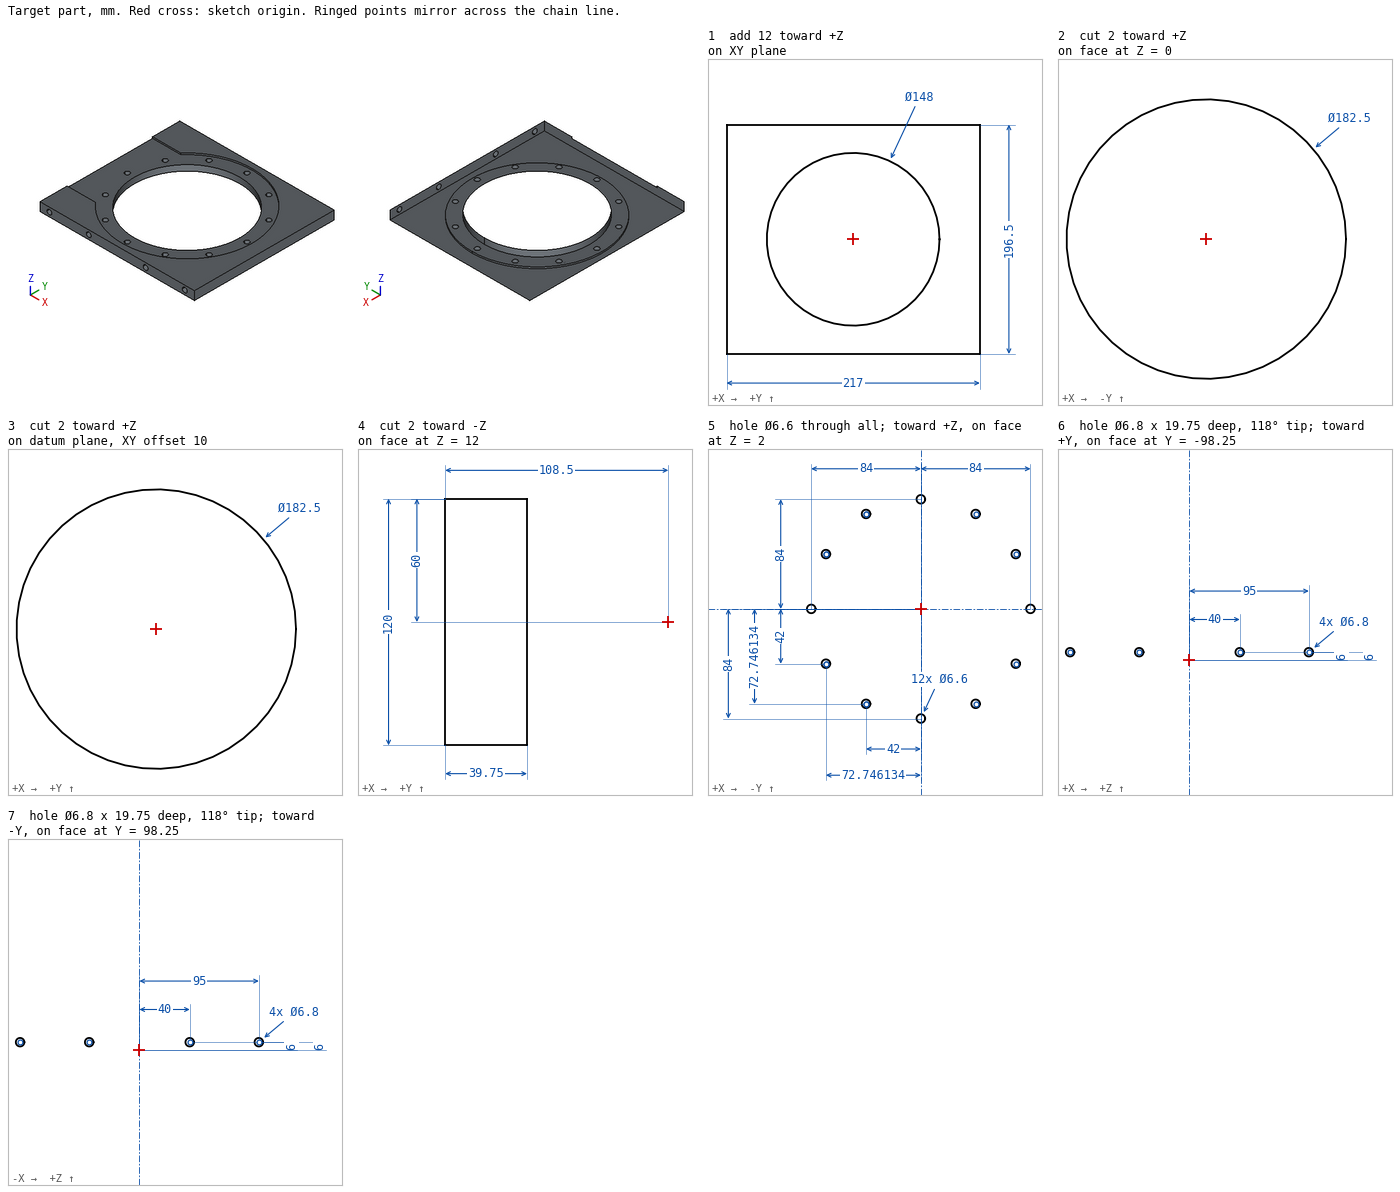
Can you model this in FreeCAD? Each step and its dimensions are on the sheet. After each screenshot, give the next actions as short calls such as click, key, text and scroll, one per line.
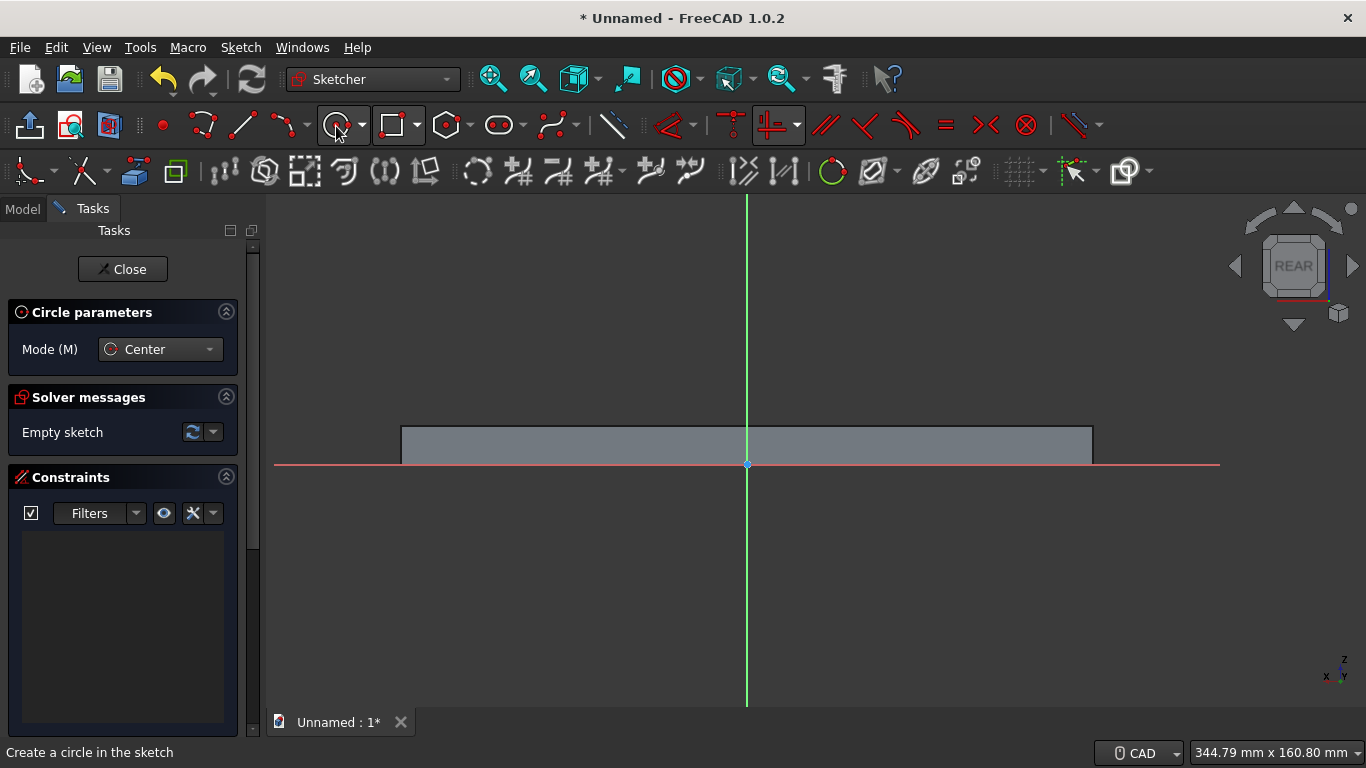
scroll(1050, 446, up, 4)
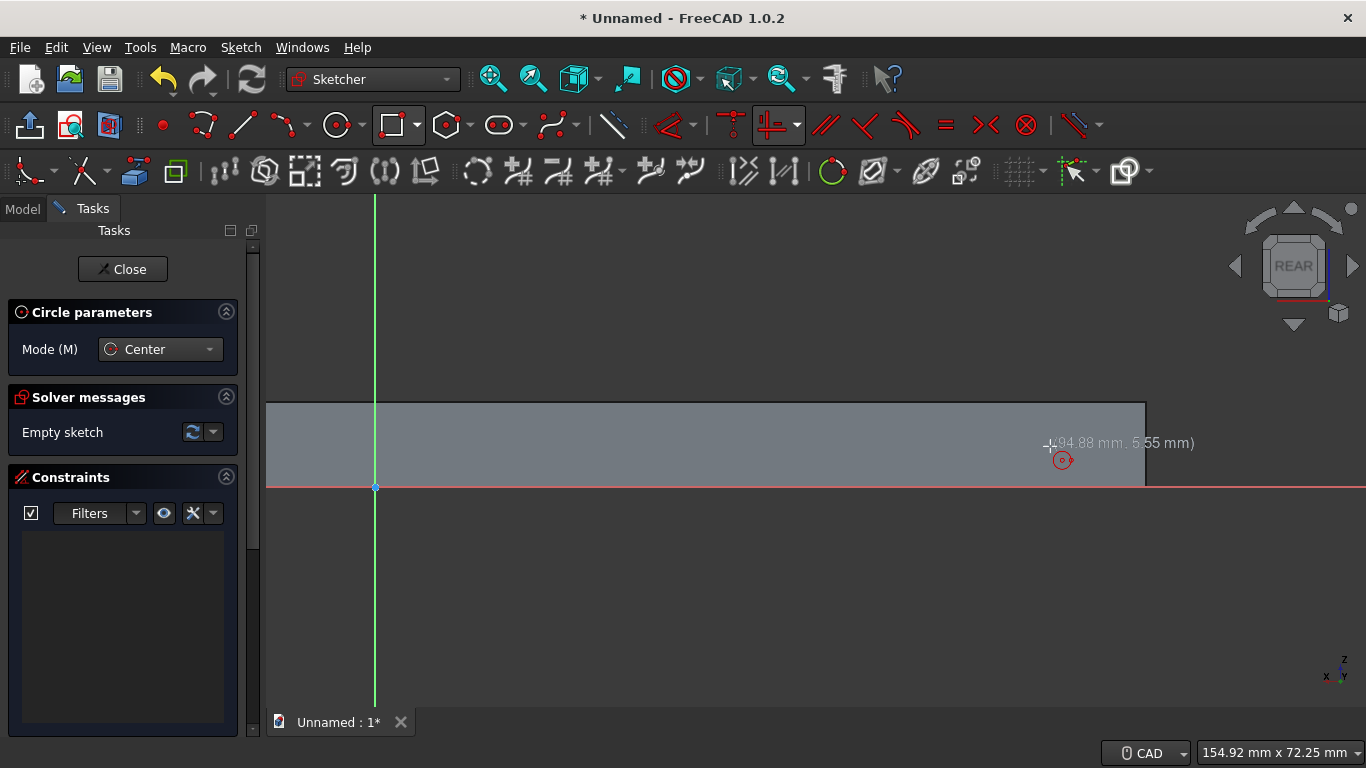
click(1050, 444)
click(1067, 427)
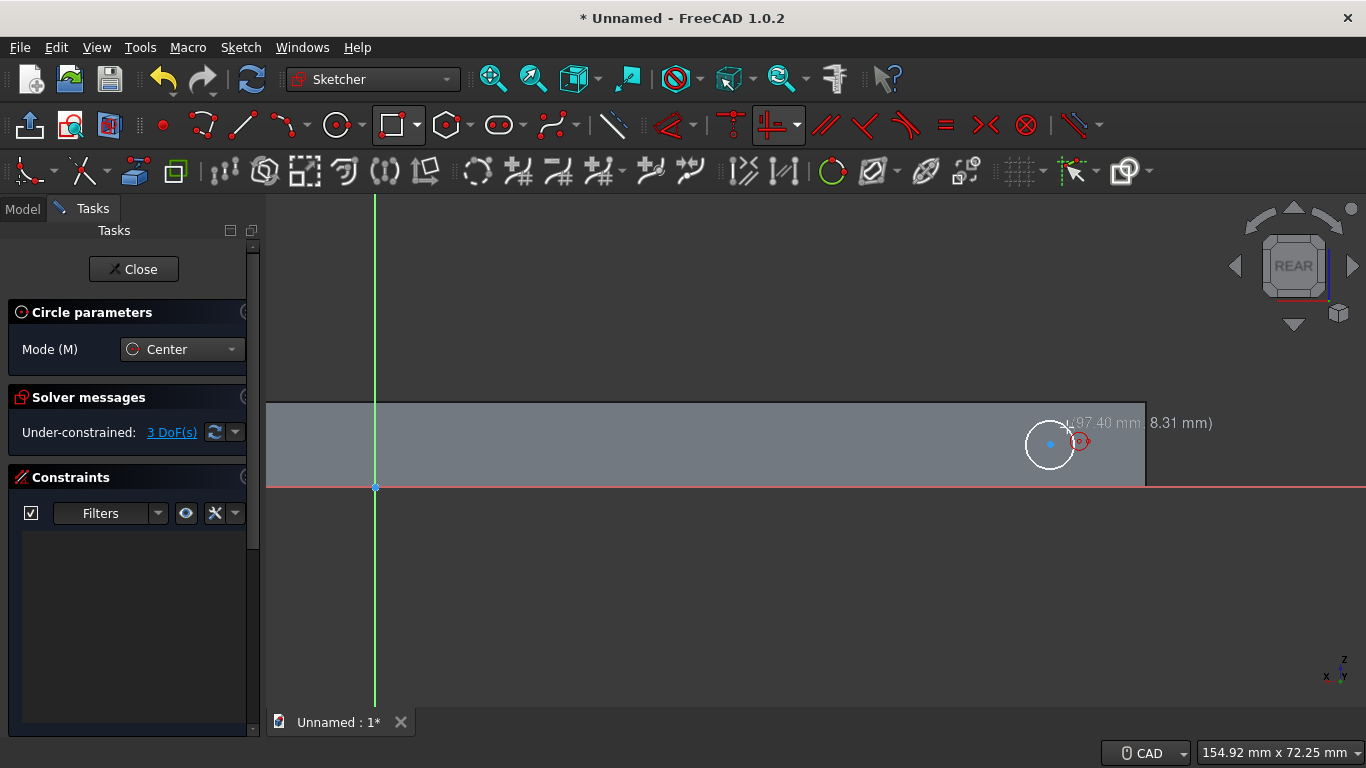
click(659, 444)
click(677, 427)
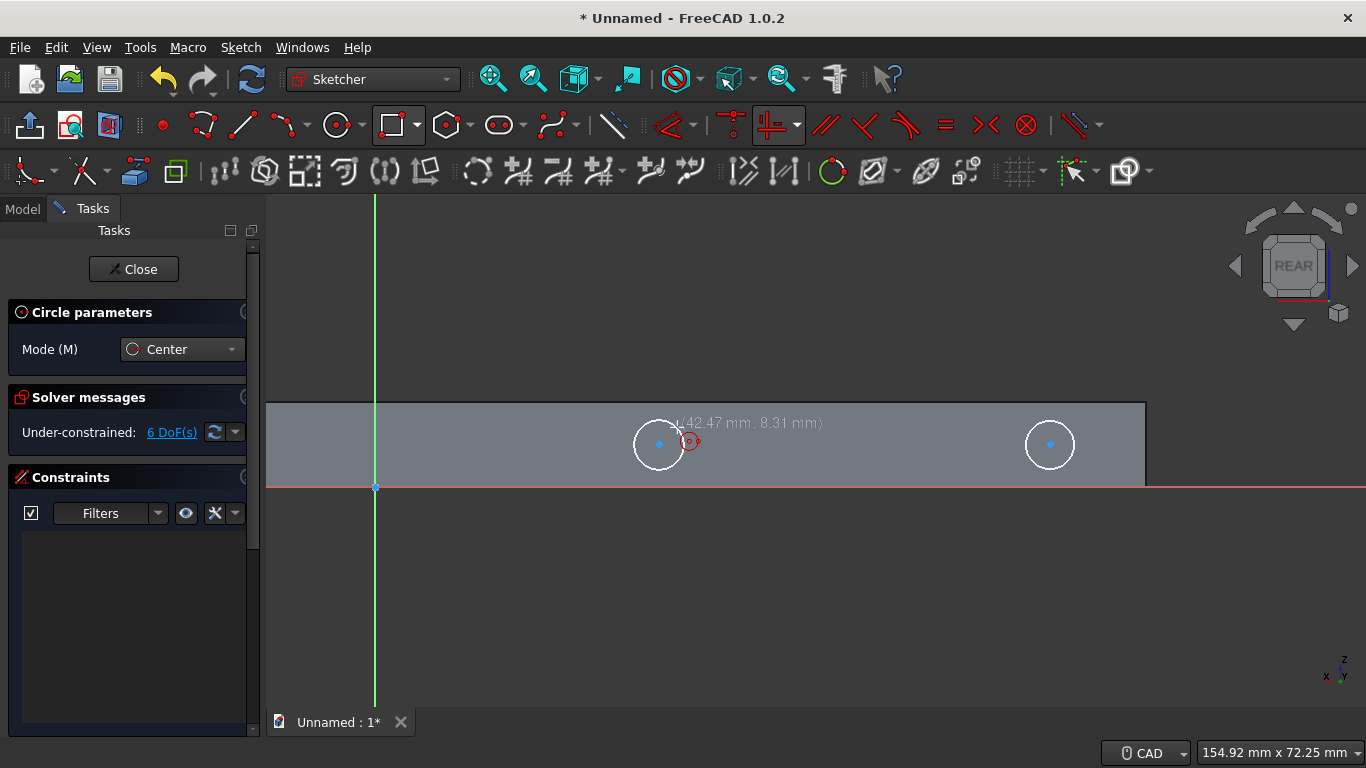
scroll(1051, 448, down, 4)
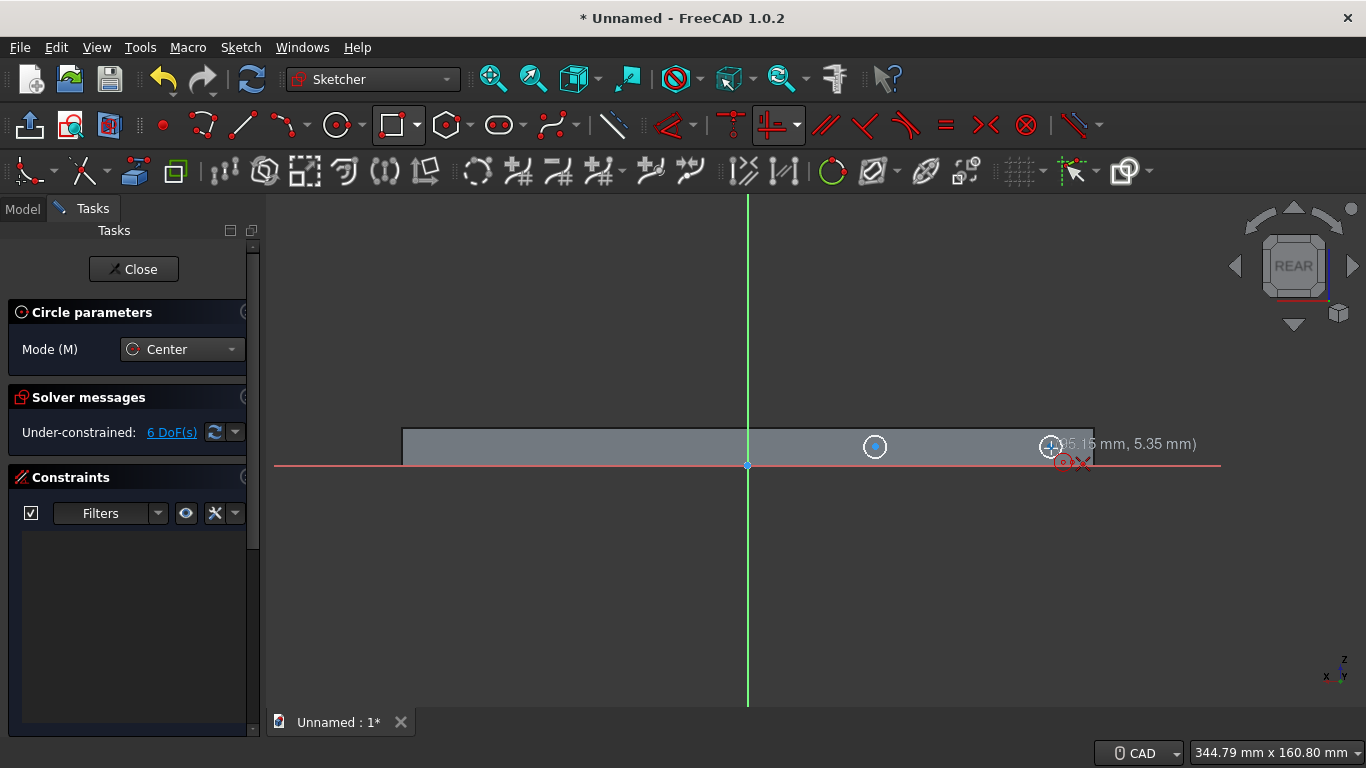
scroll(620, 447, up, 4)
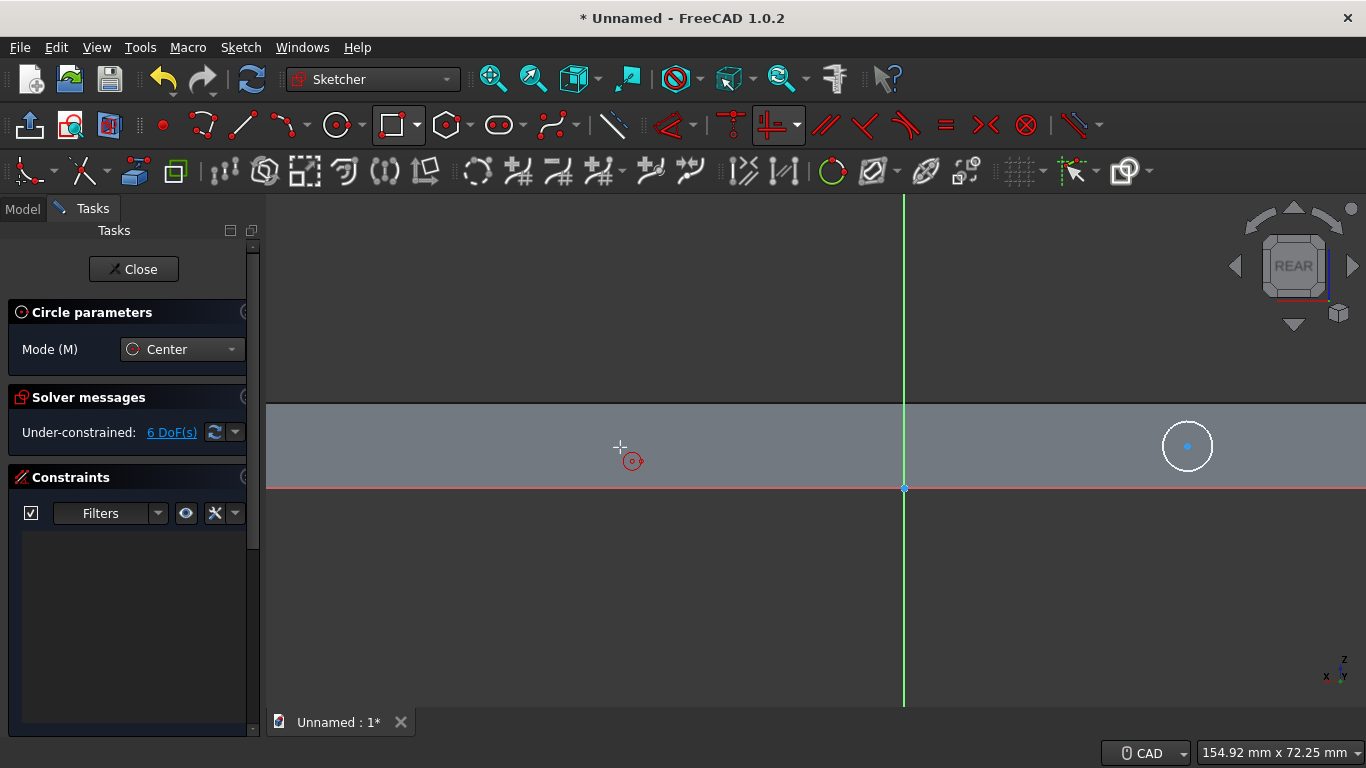
click(620, 446)
click(637, 429)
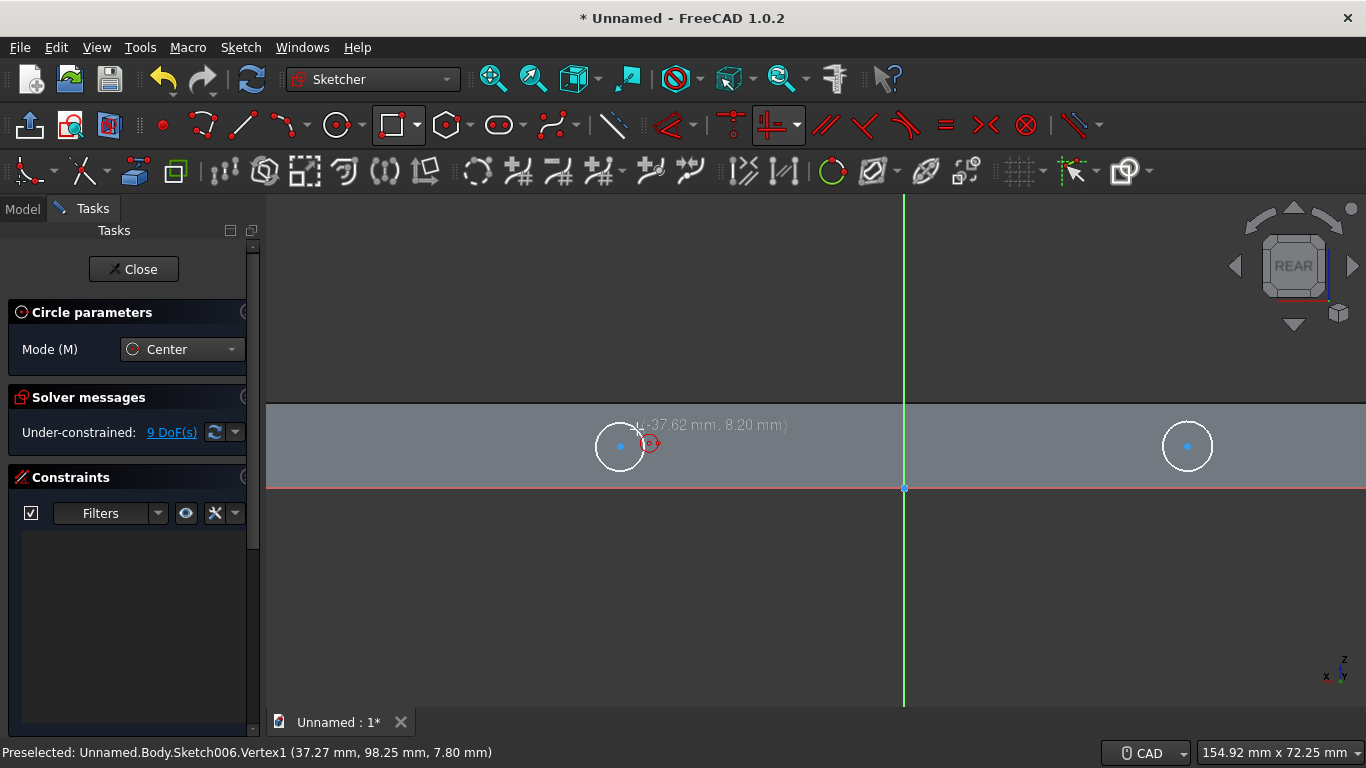
scroll(620, 447, down, 4)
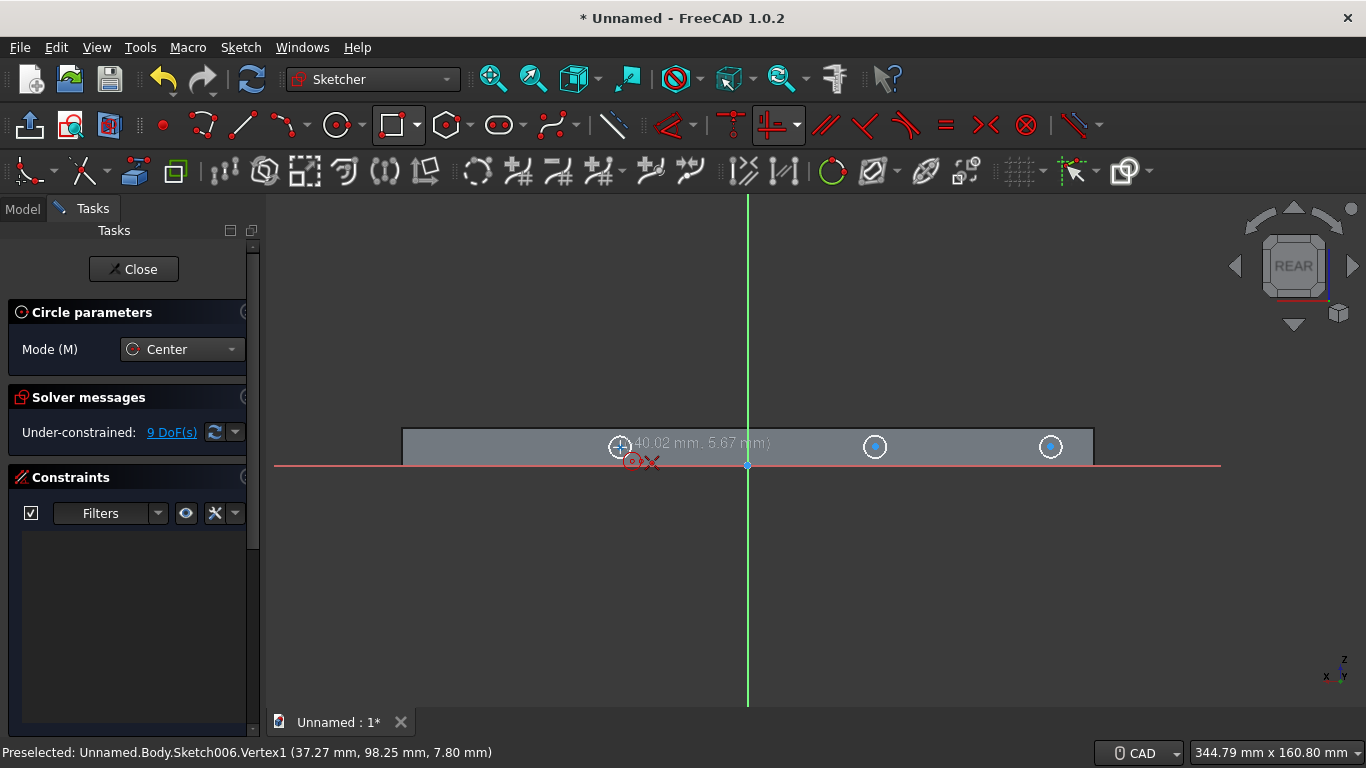
scroll(445, 447, up, 4)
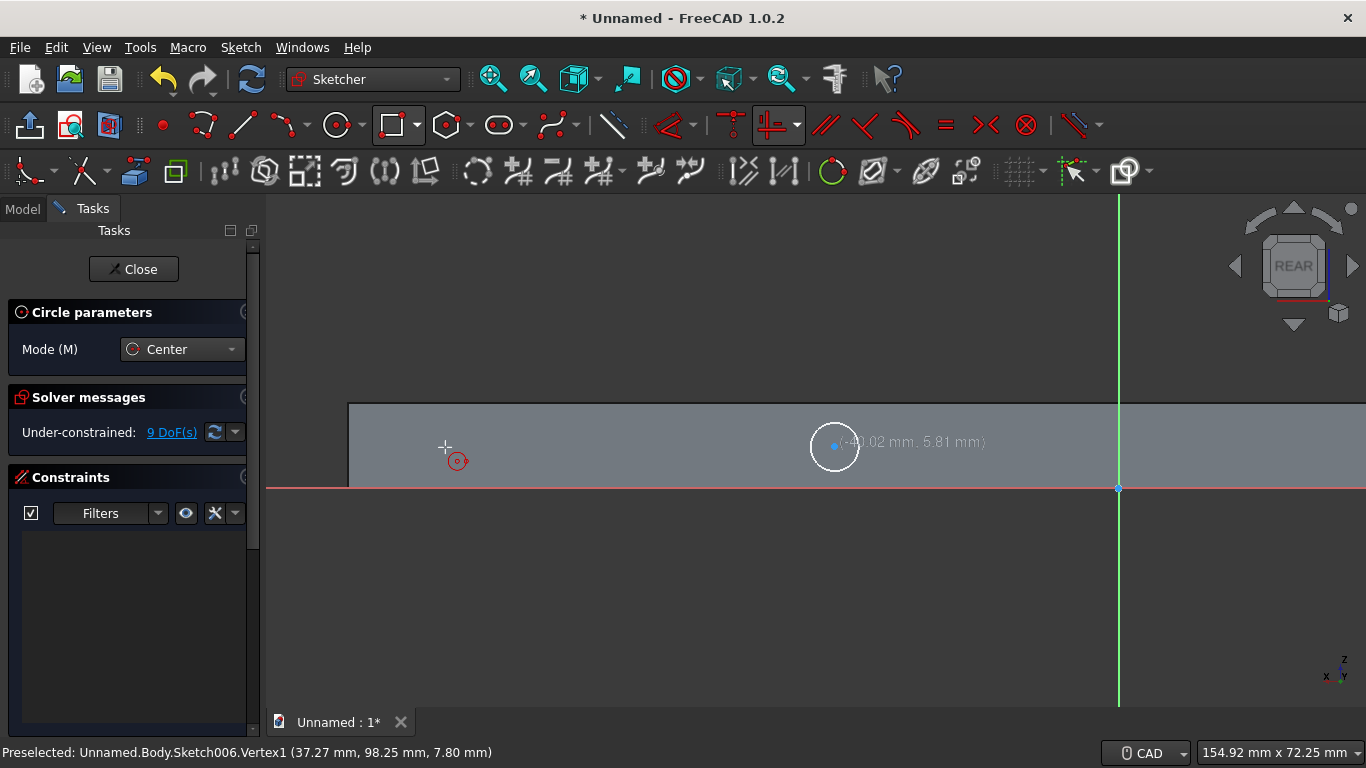
click(444, 446)
click(461, 429)
key(Escape)